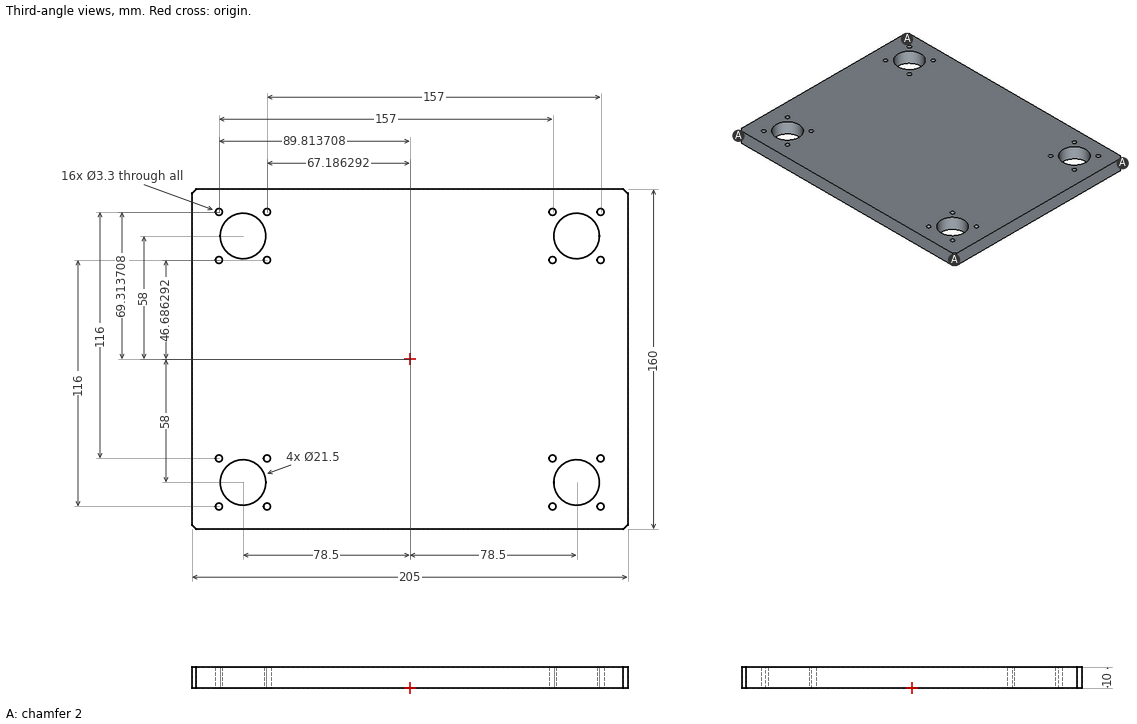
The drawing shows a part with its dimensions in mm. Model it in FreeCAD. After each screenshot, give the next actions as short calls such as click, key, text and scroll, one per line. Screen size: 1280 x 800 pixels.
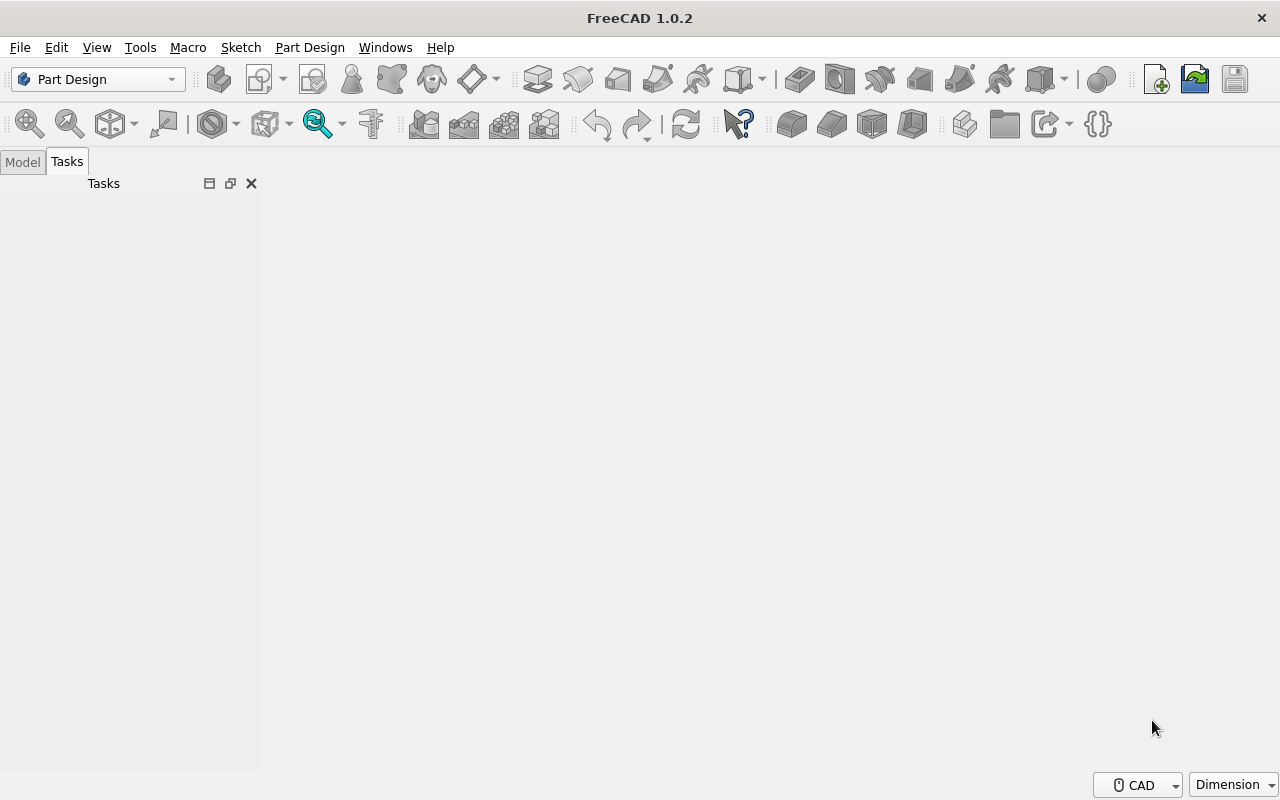
key(ctrl+n)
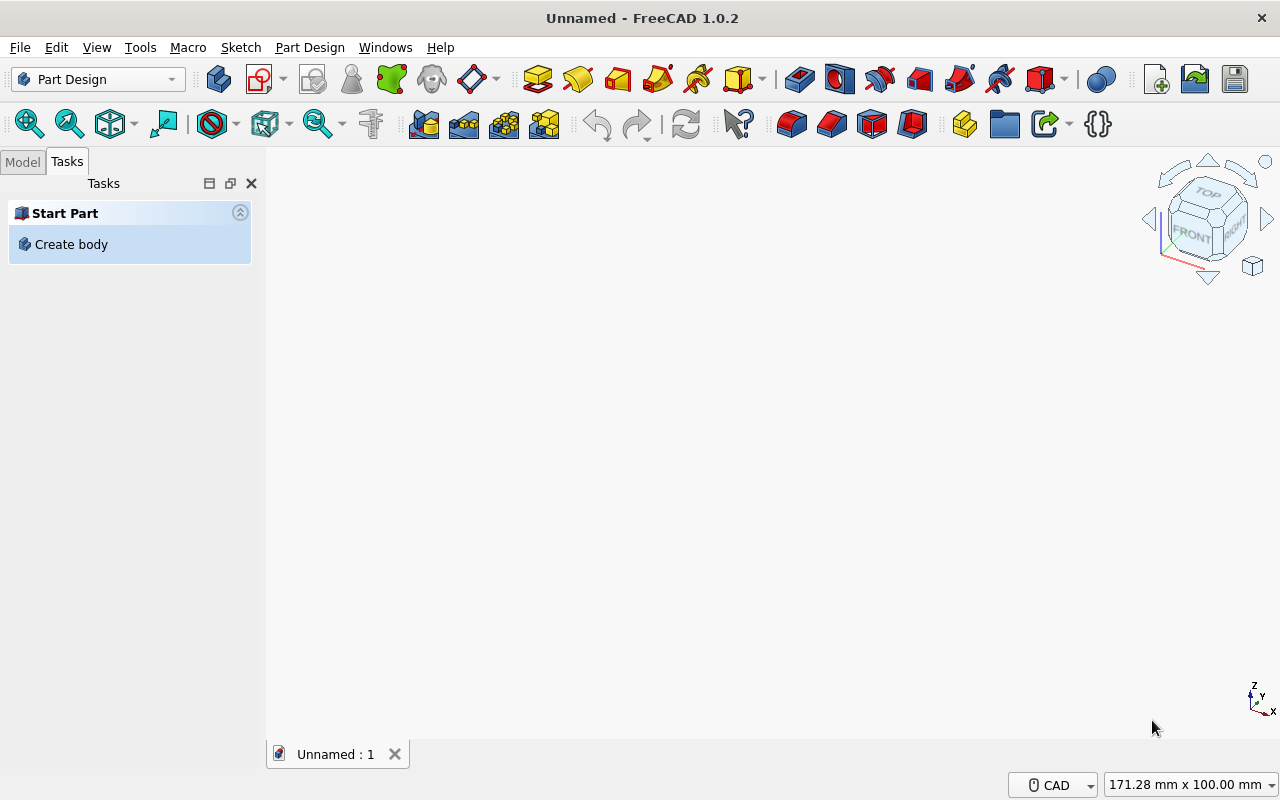
click(260, 80)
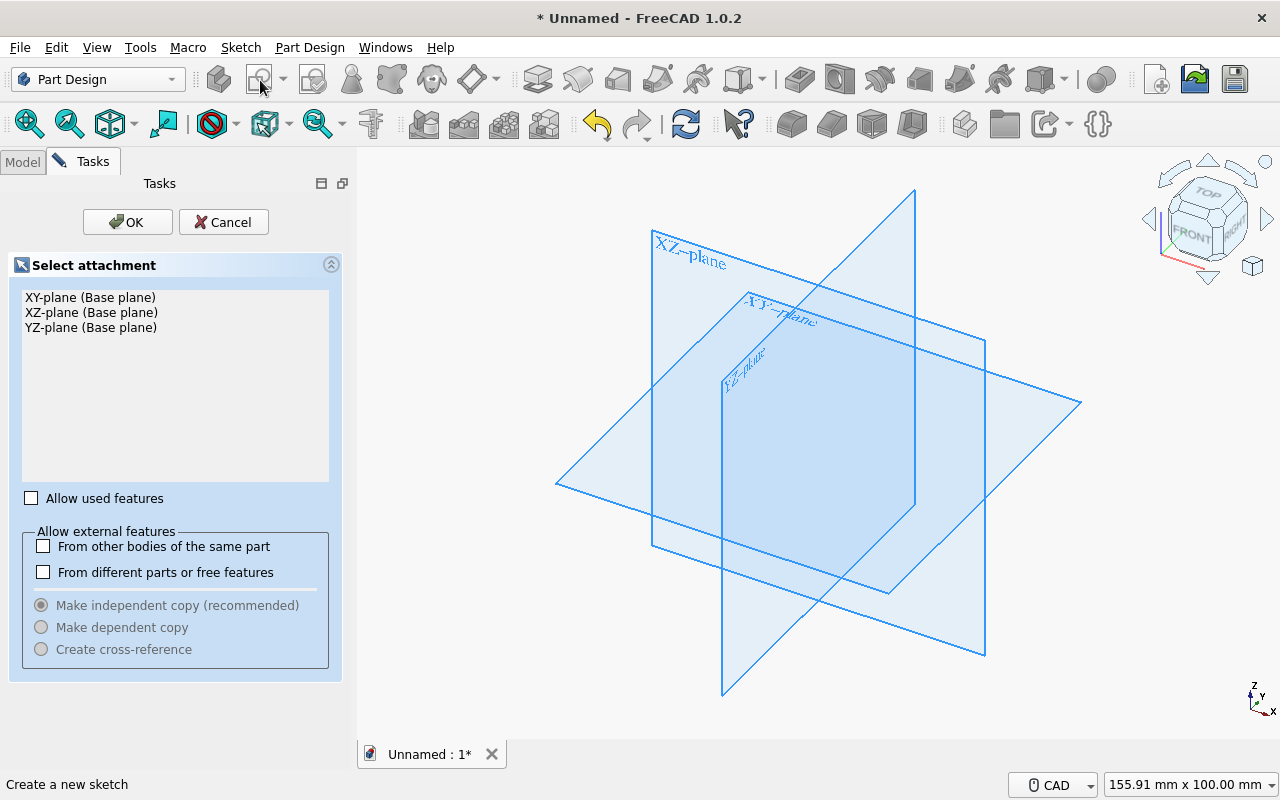
click(82, 298)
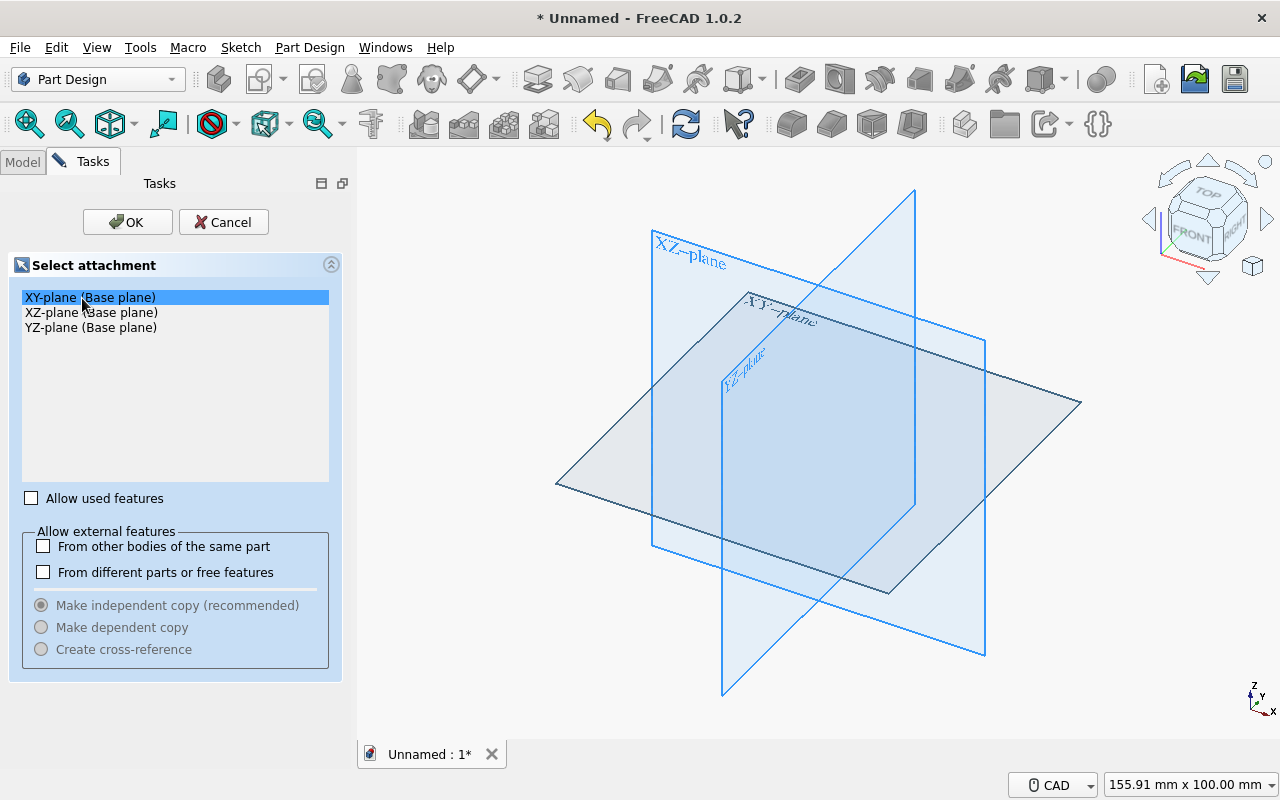
click(128, 222)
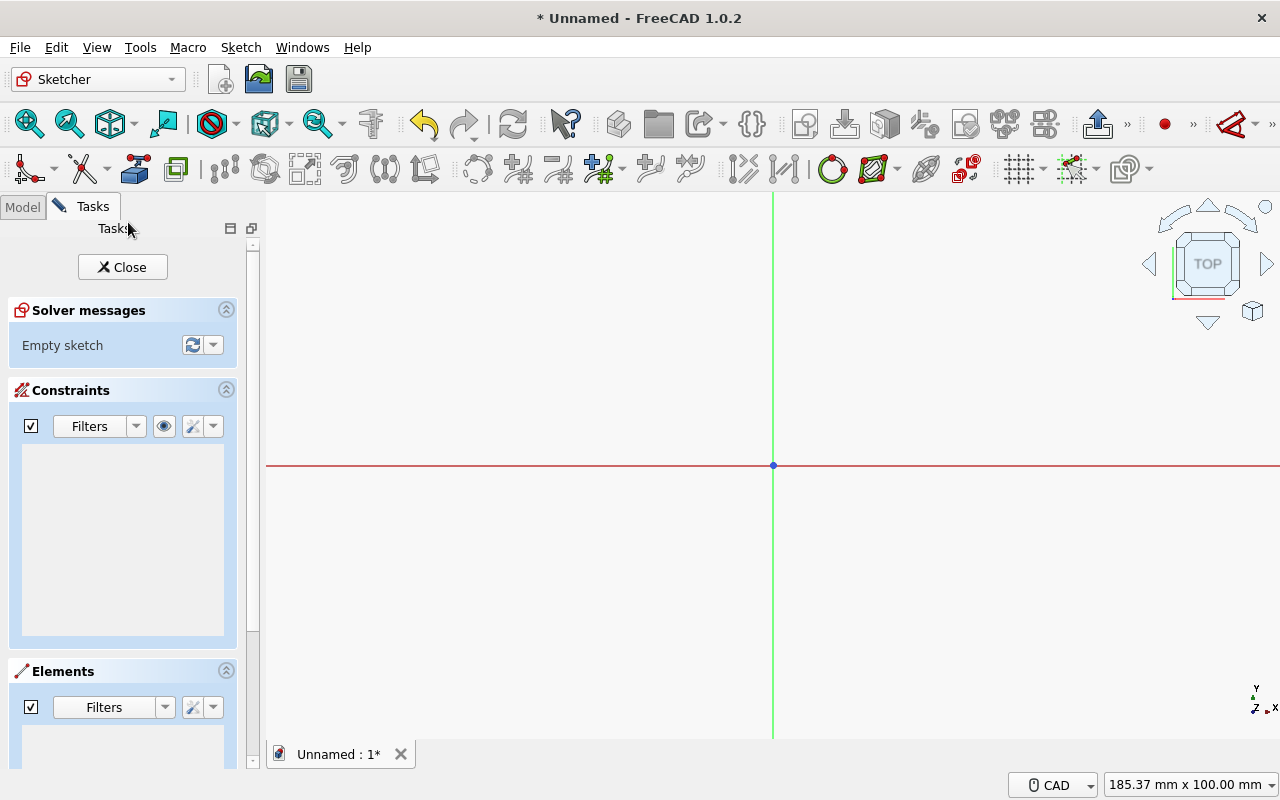
scroll(665, 466, down, 5)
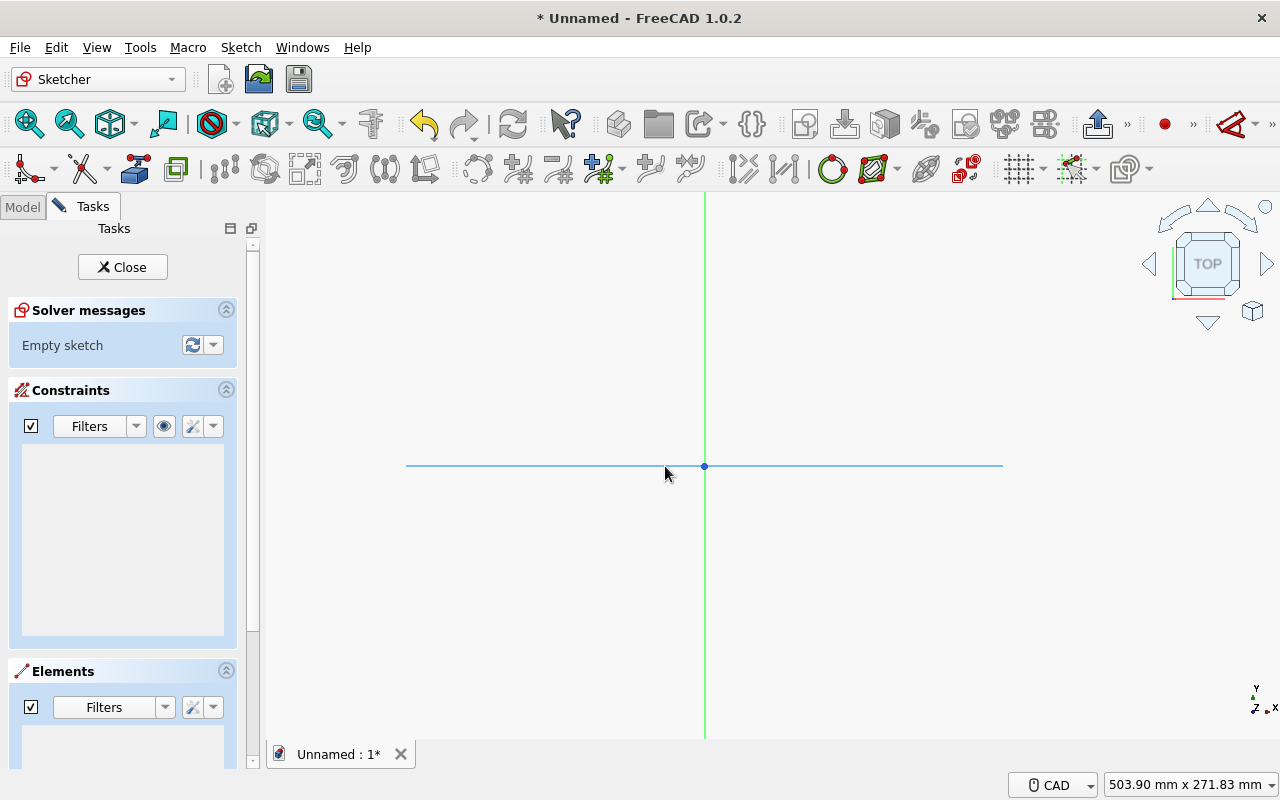
key(g)
key(v)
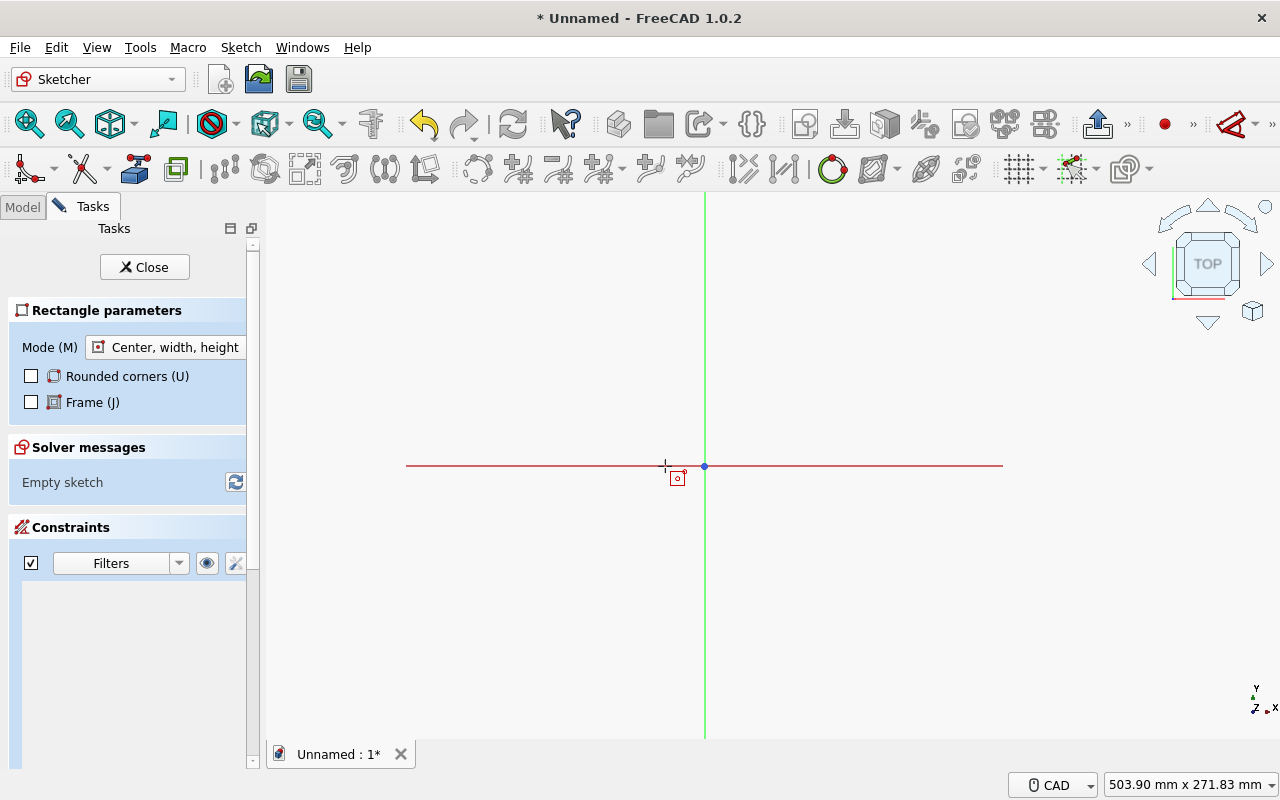
click(705, 466)
move(911, 305)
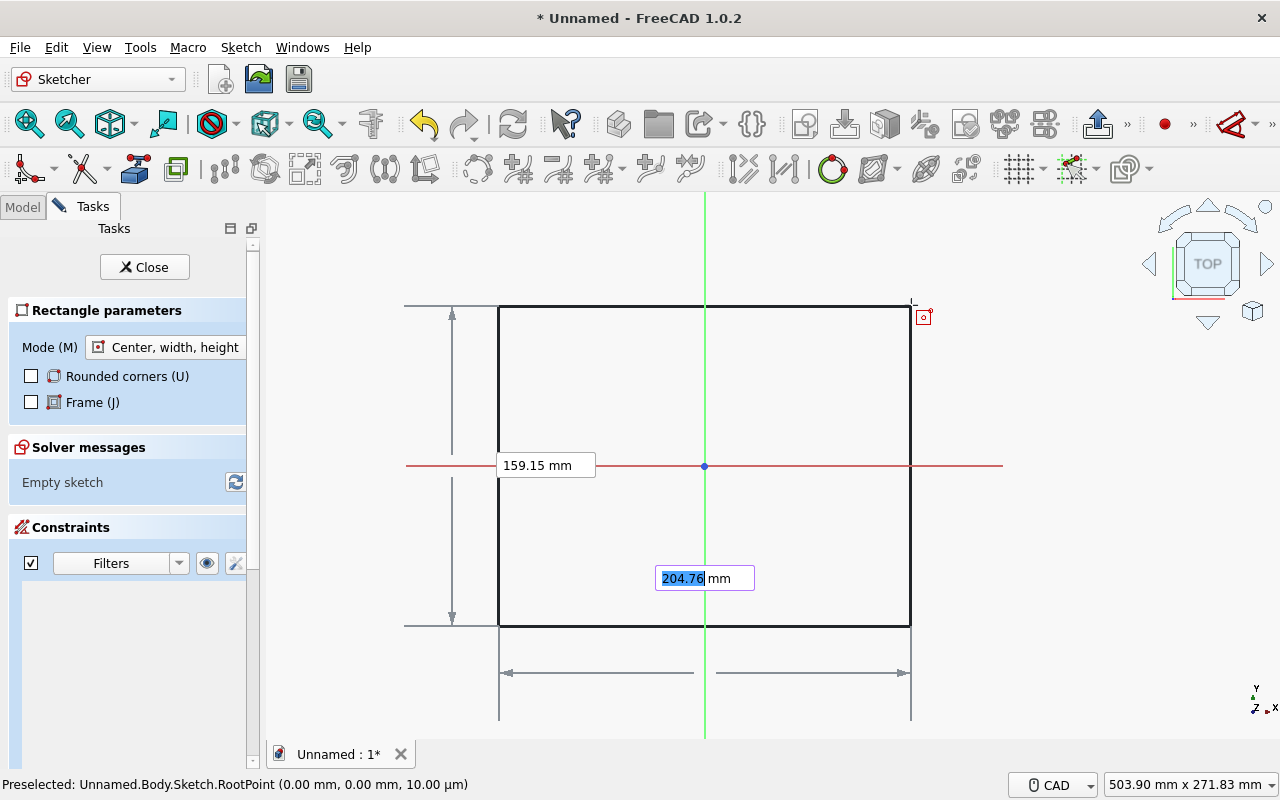
text(205)
key(Tab)
text(160)
key(Return)
key(Escape)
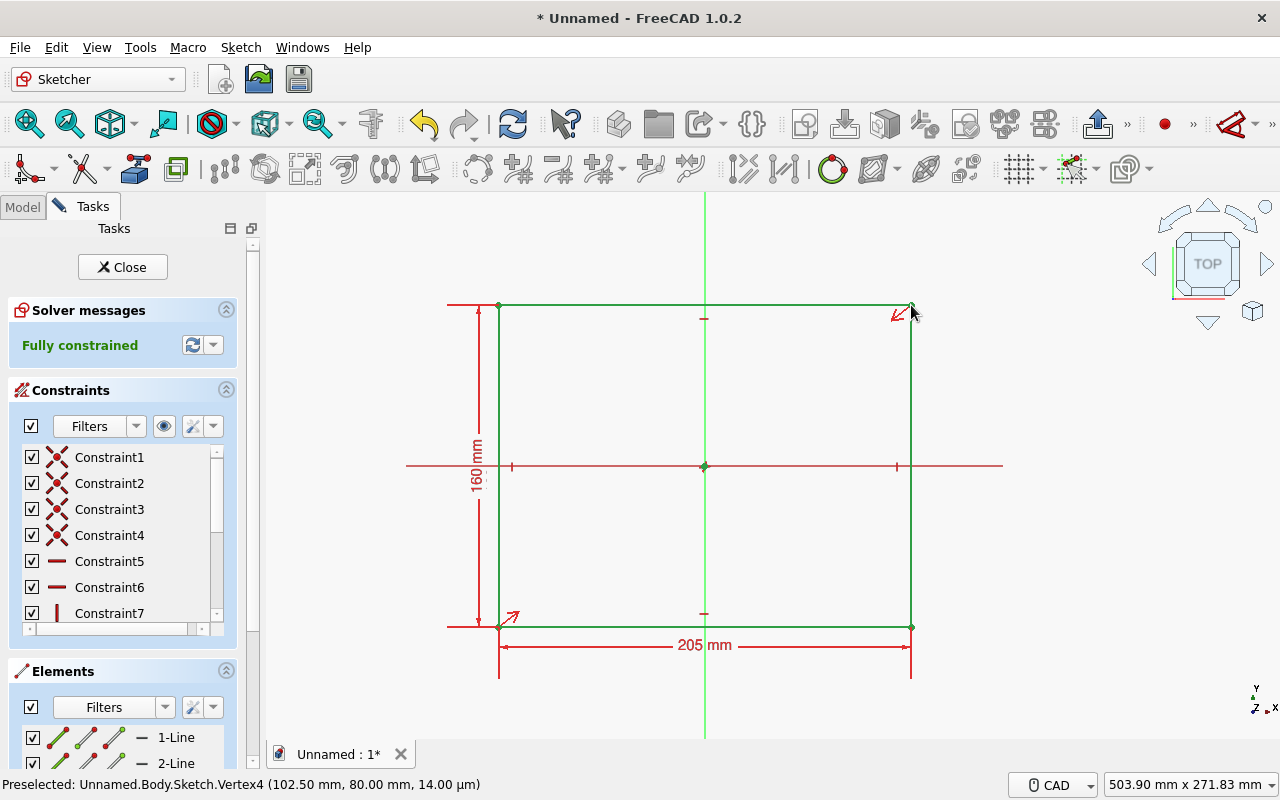
click(123, 267)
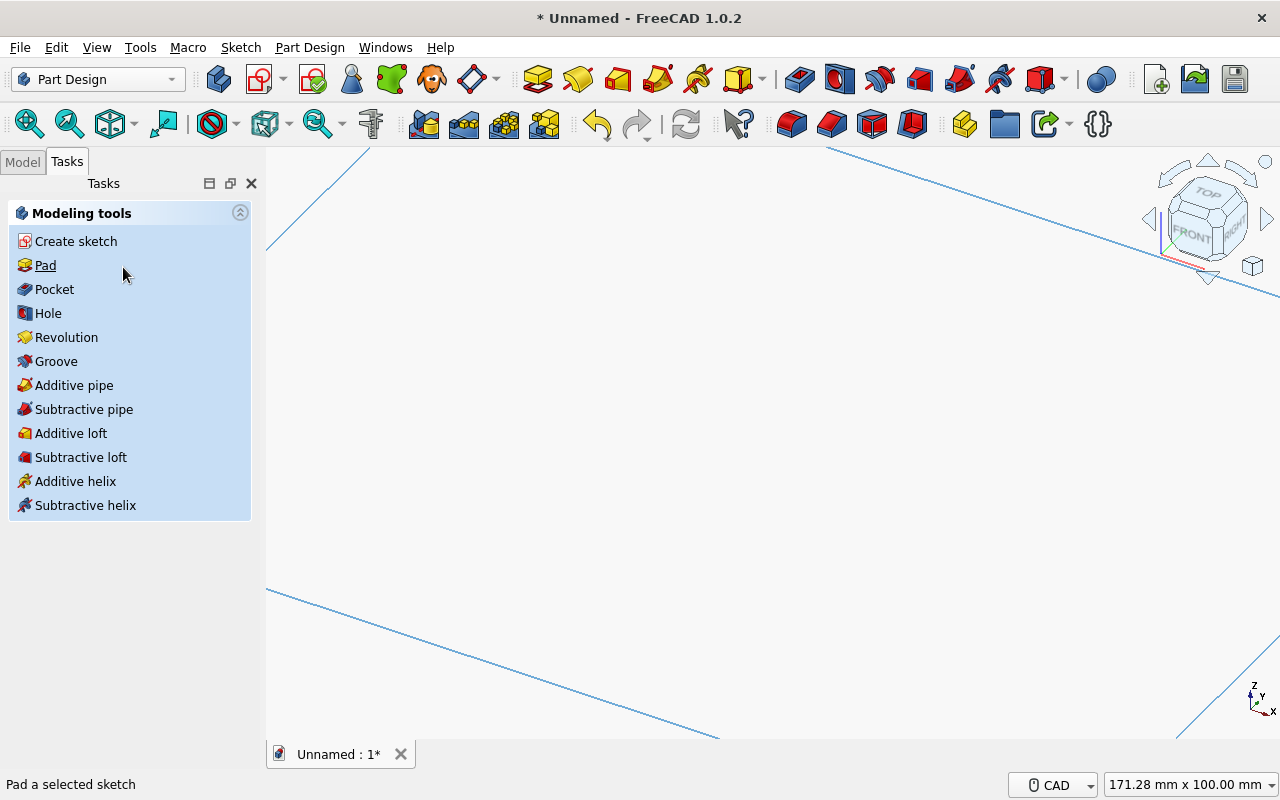
click(538, 80)